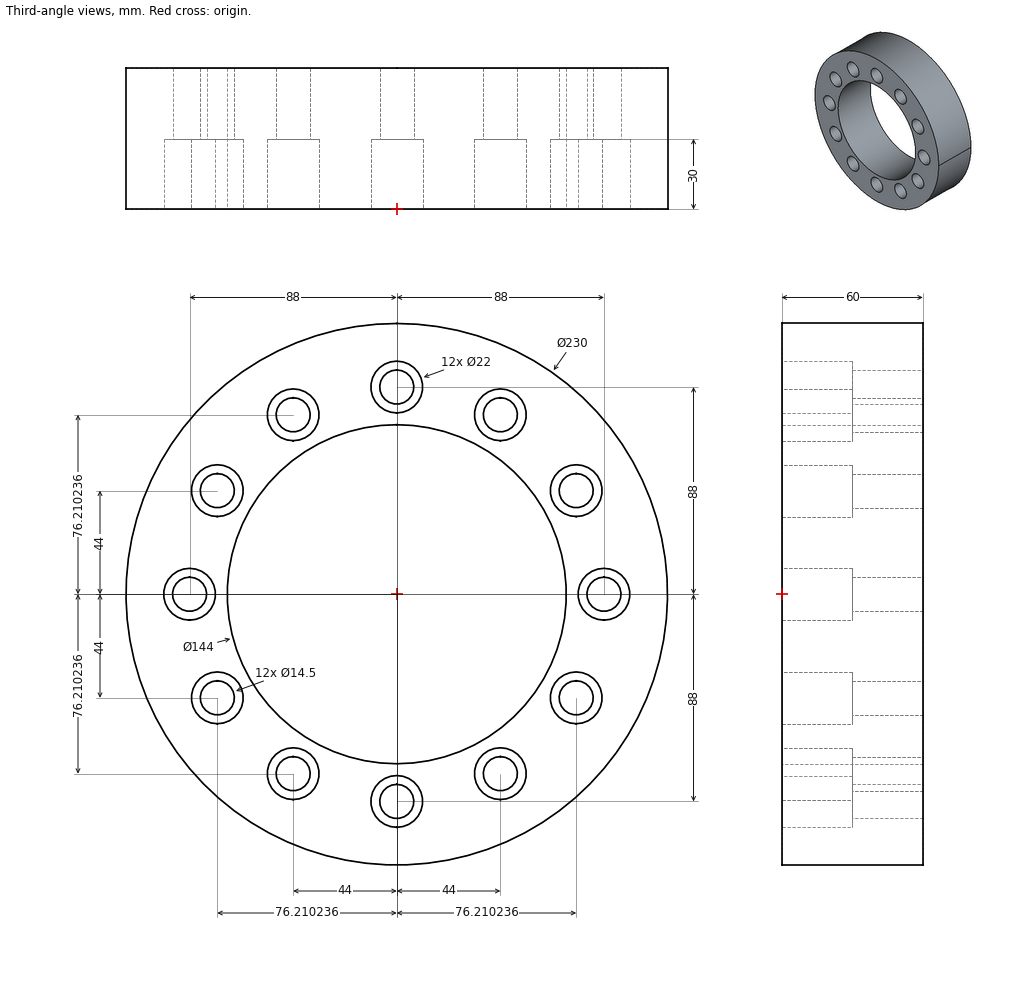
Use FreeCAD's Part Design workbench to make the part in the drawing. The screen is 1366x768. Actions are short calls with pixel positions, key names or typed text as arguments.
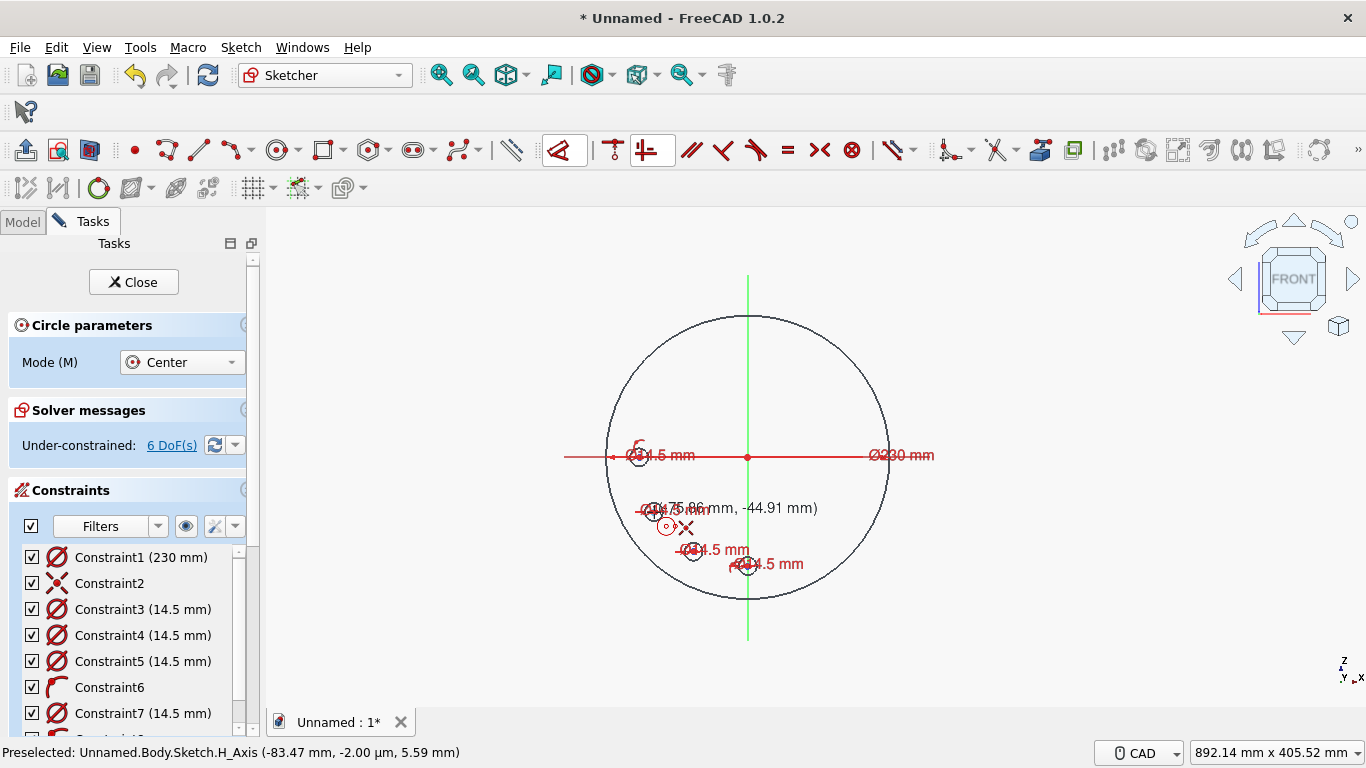
scroll(654, 403, up, 5)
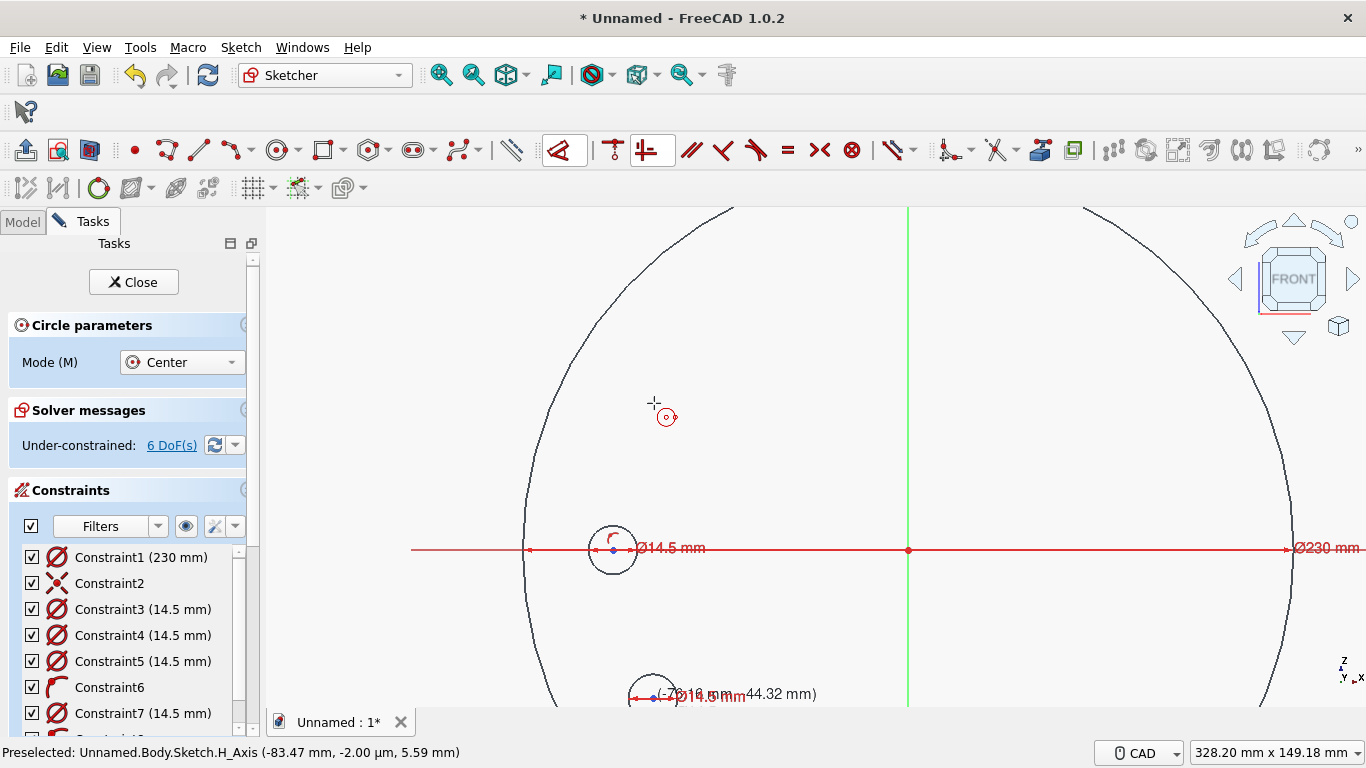
click(653, 403)
move(670, 385)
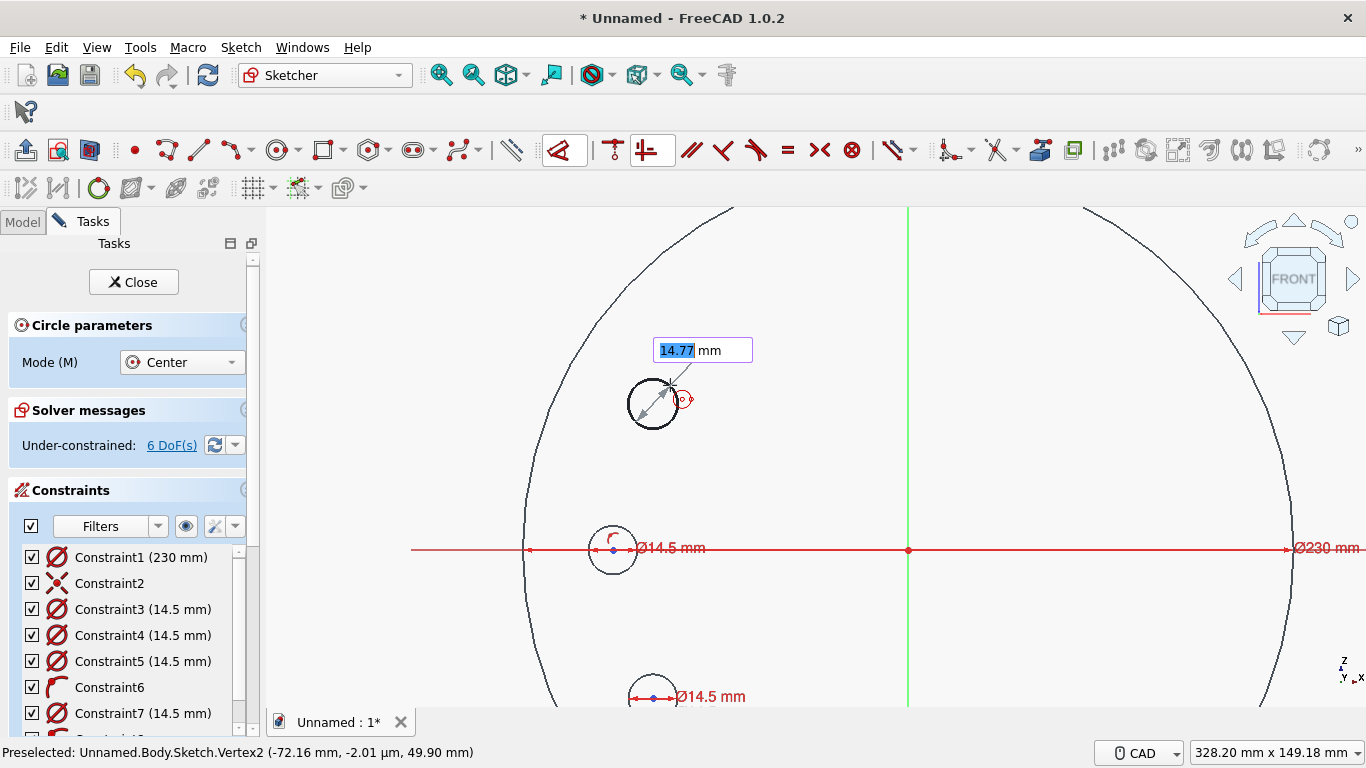
text(14.5)
key(Return)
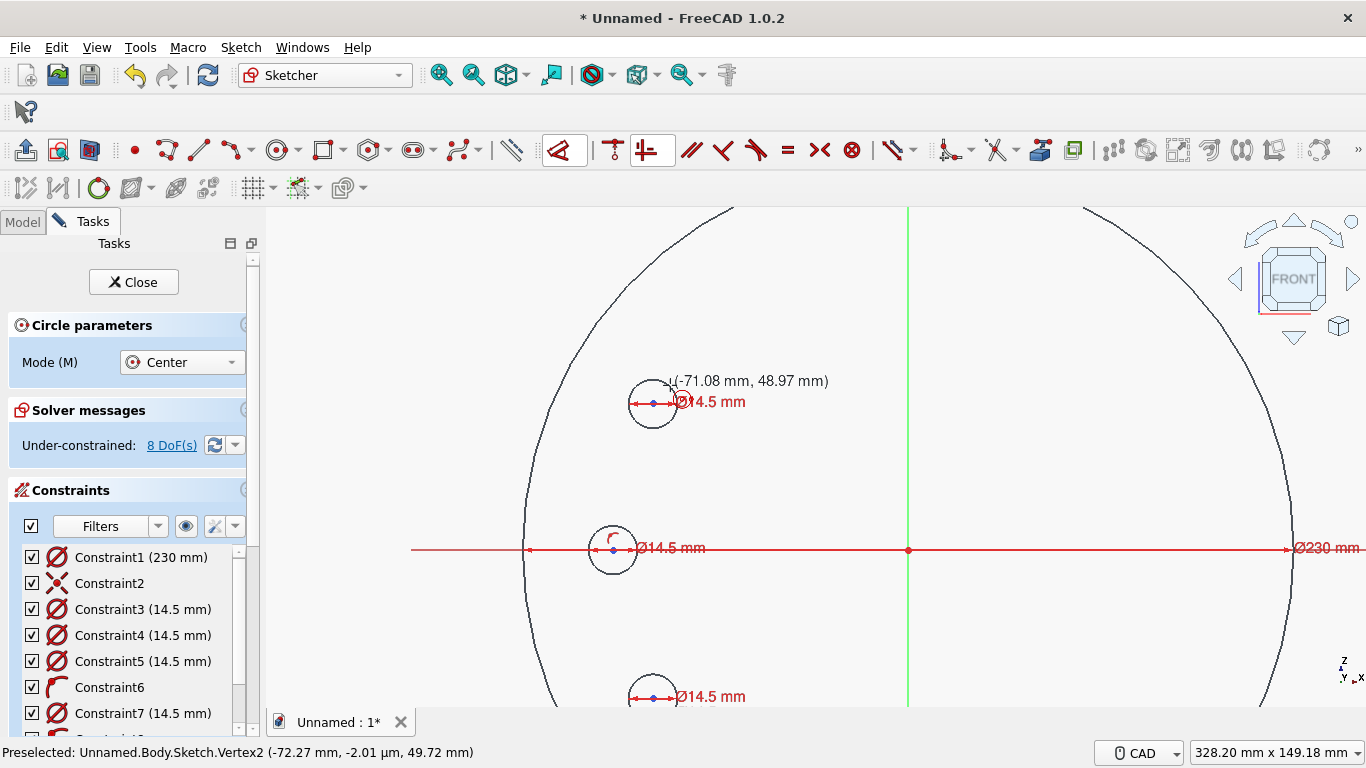
click(761, 295)
move(778, 278)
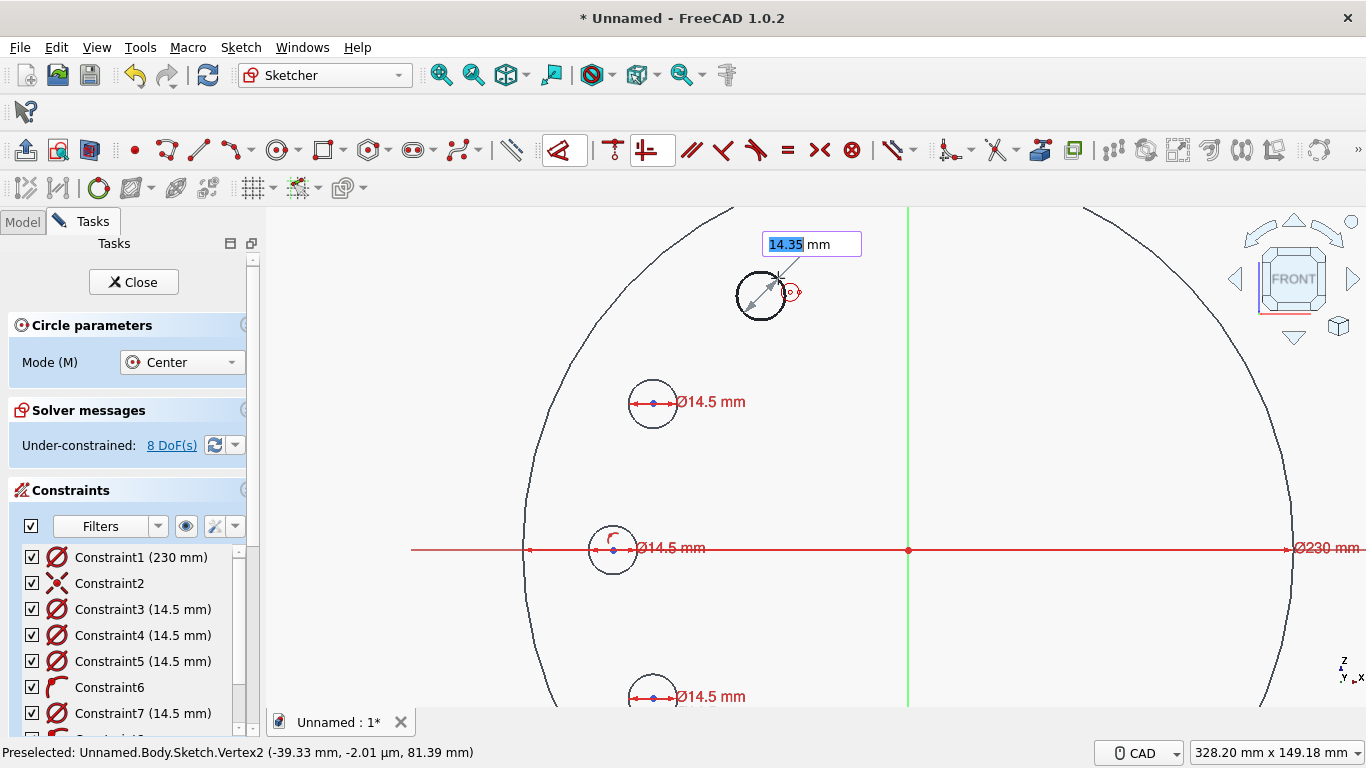
text(14.5)
key(Return)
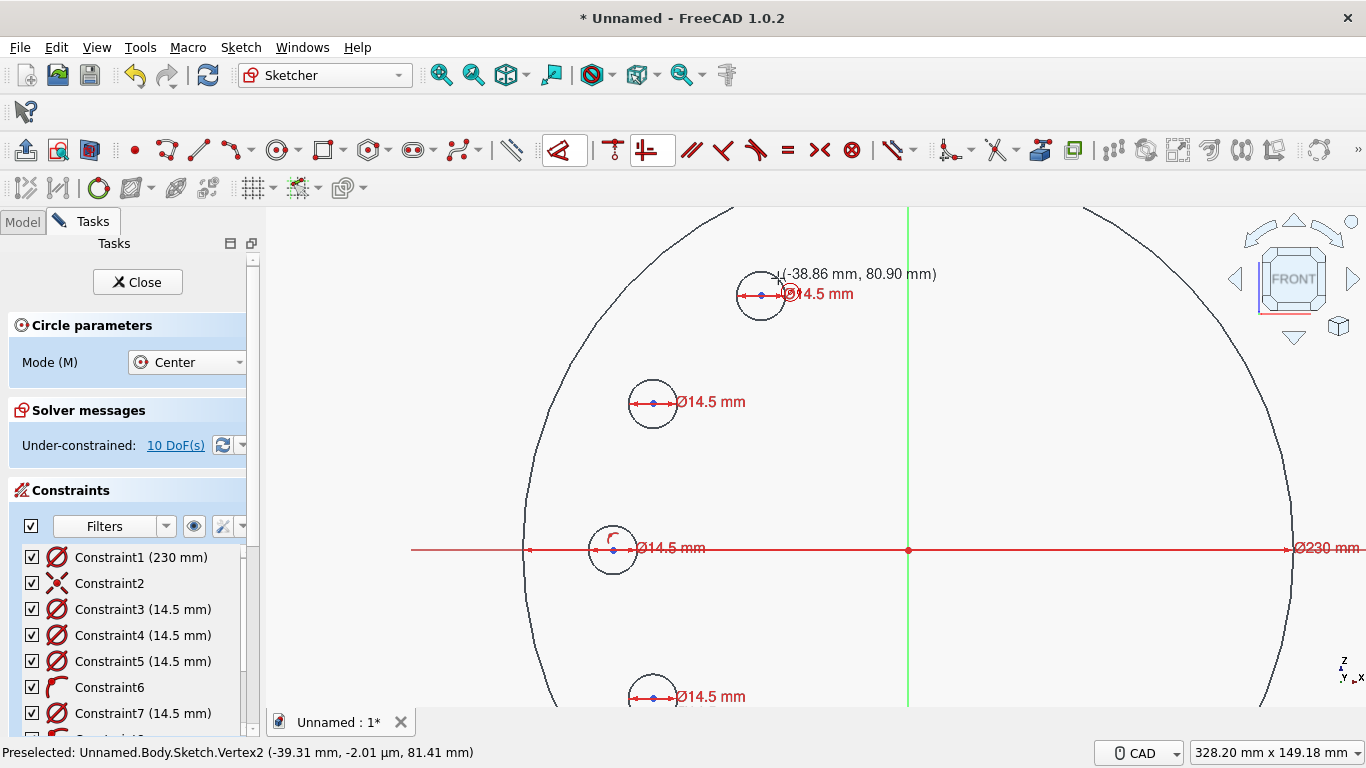
scroll(654, 403, down, 5)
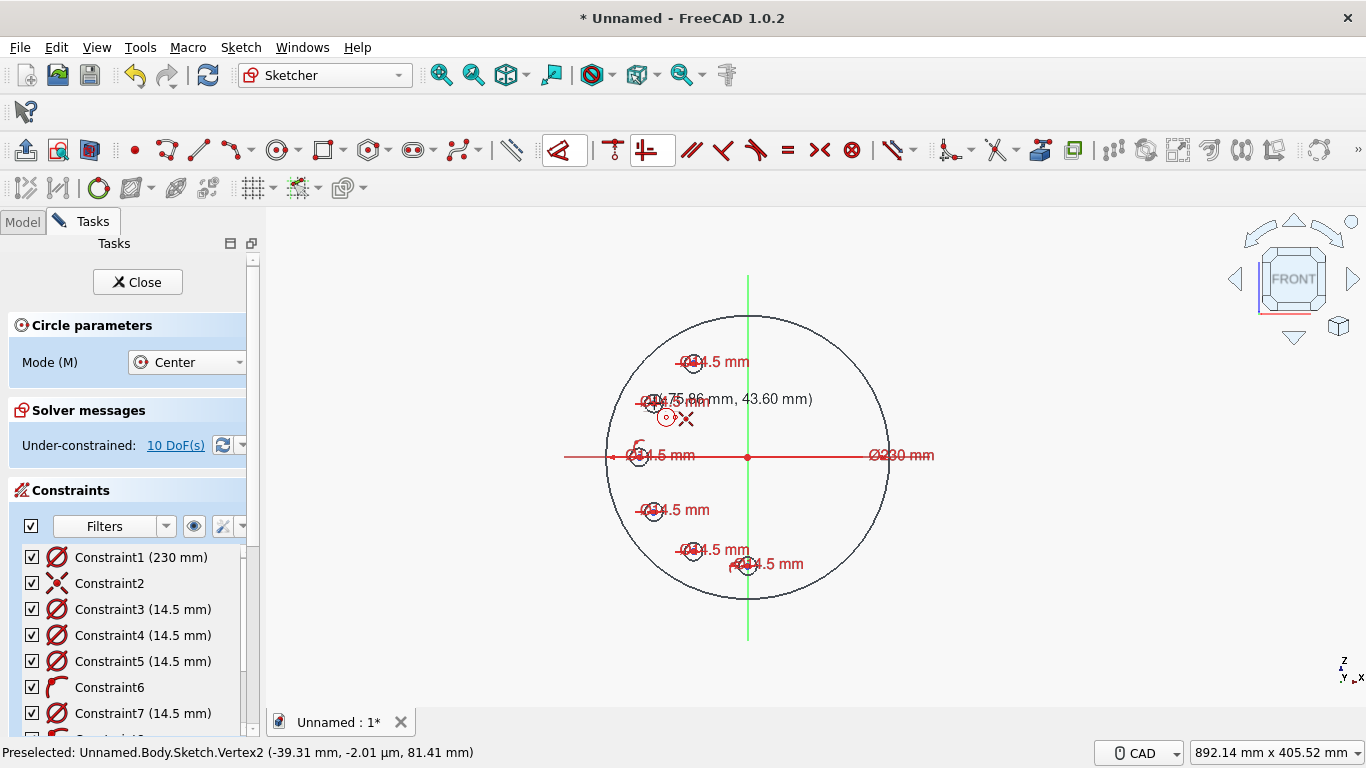
scroll(802, 551, up, 5)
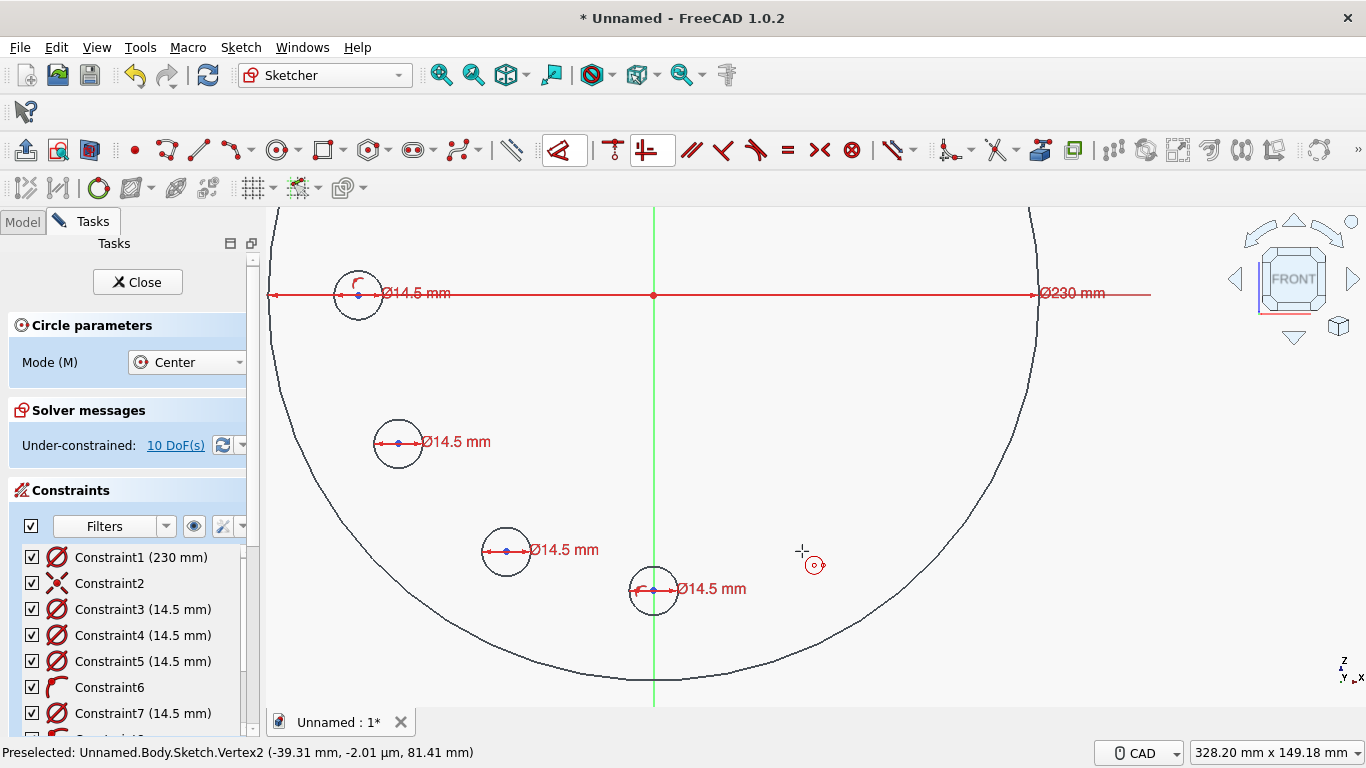
click(801, 551)
move(818, 534)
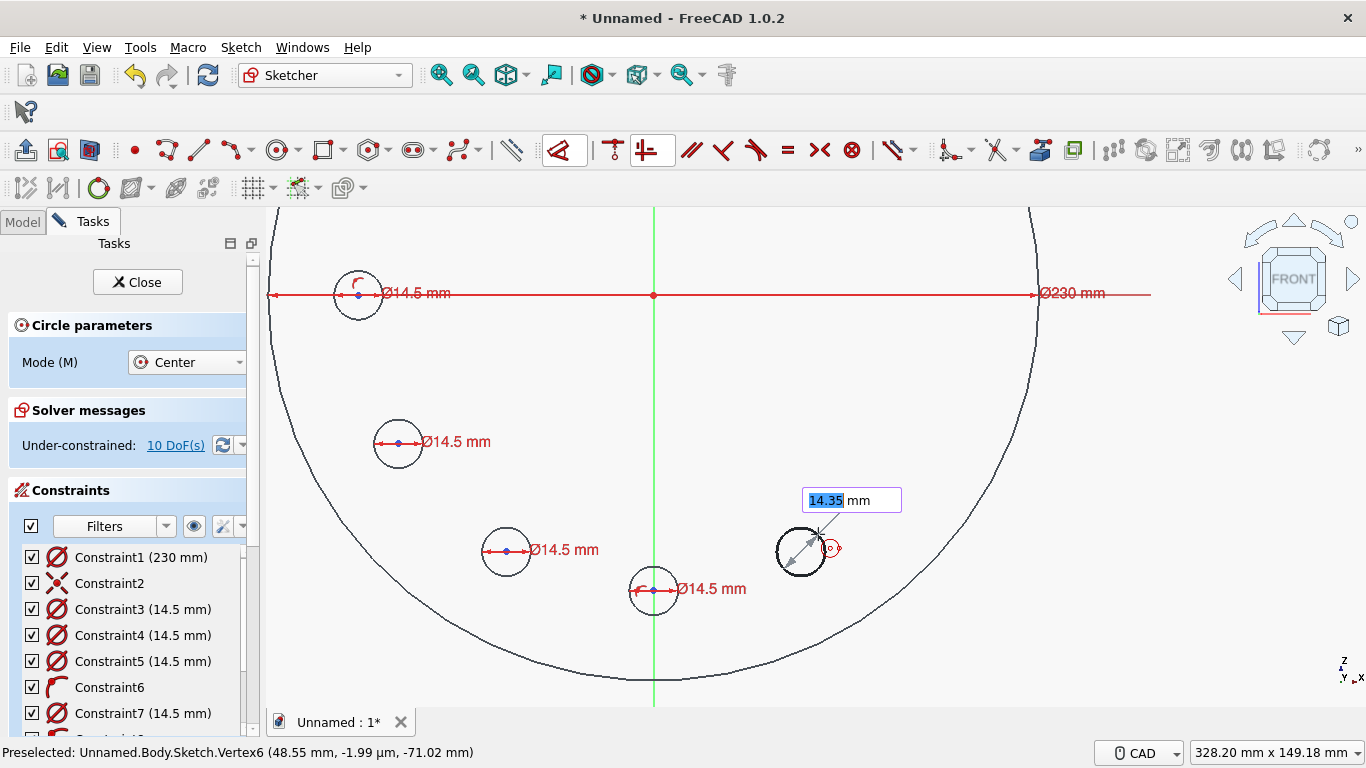
text(14.5)
key(Return)